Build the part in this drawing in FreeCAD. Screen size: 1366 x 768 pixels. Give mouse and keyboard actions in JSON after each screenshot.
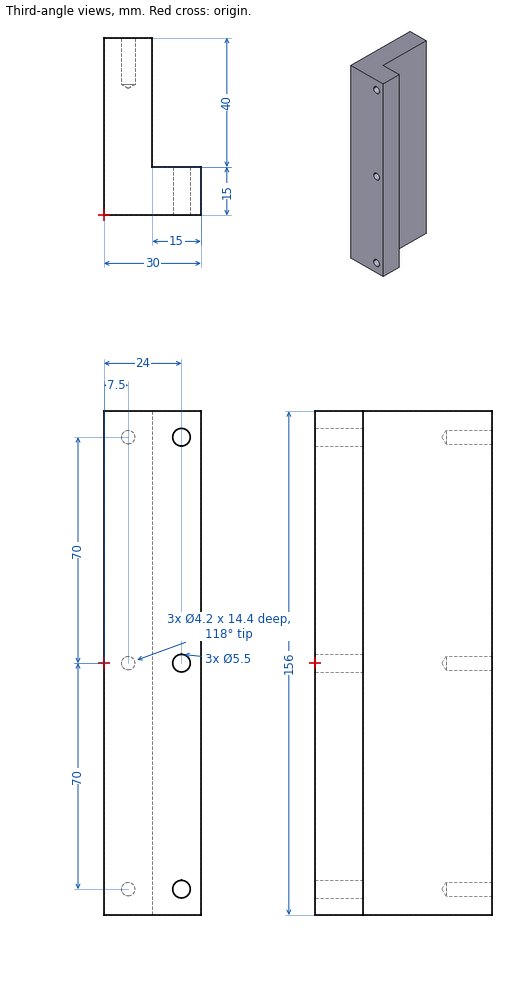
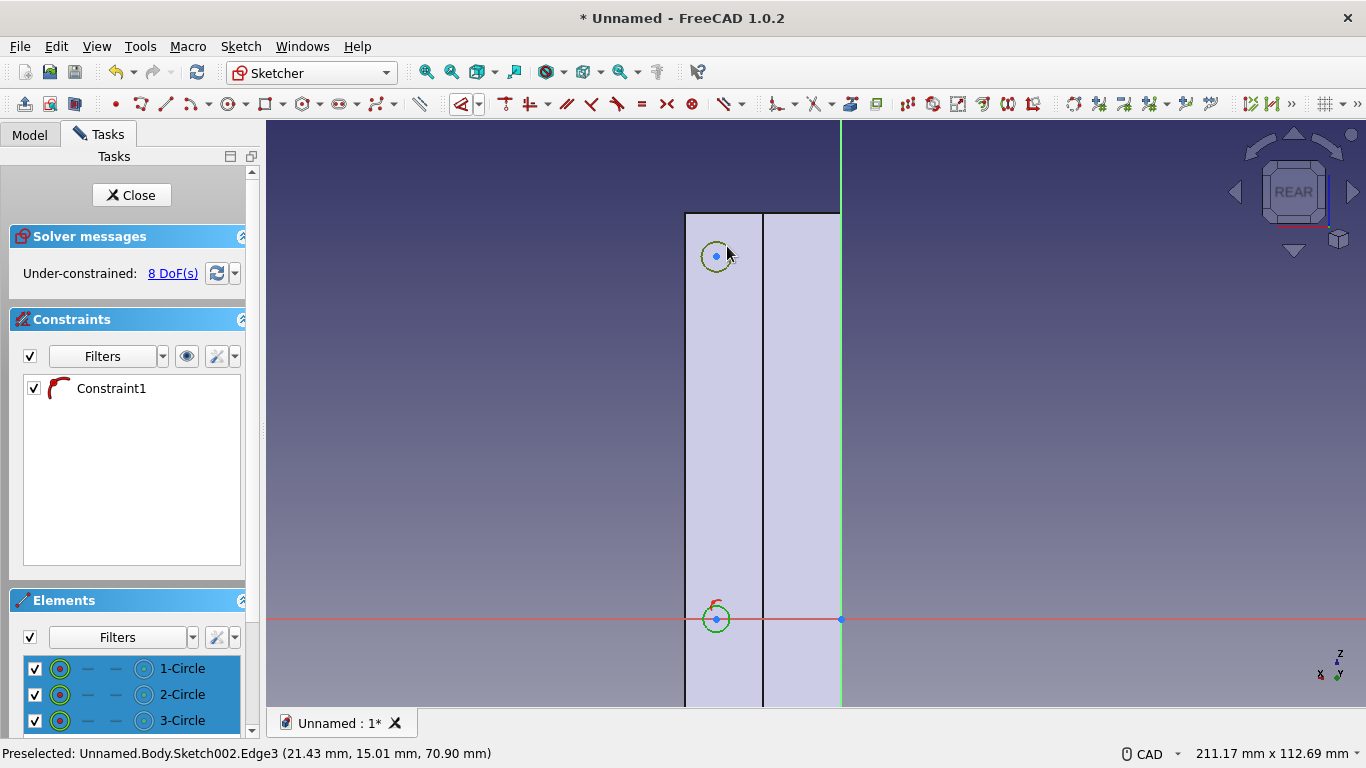
{"action": "key", "text": "e"}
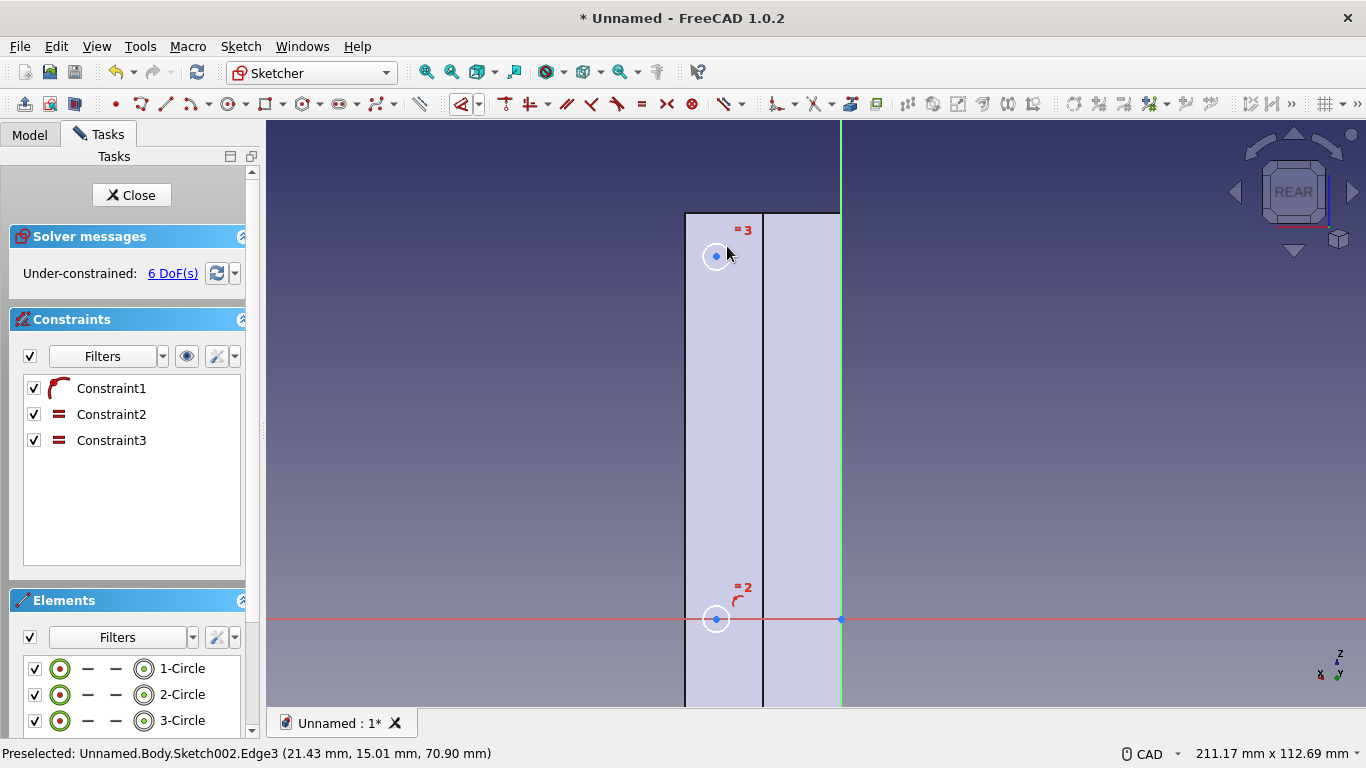
{"action": "left_click", "coordinate": [716, 619]}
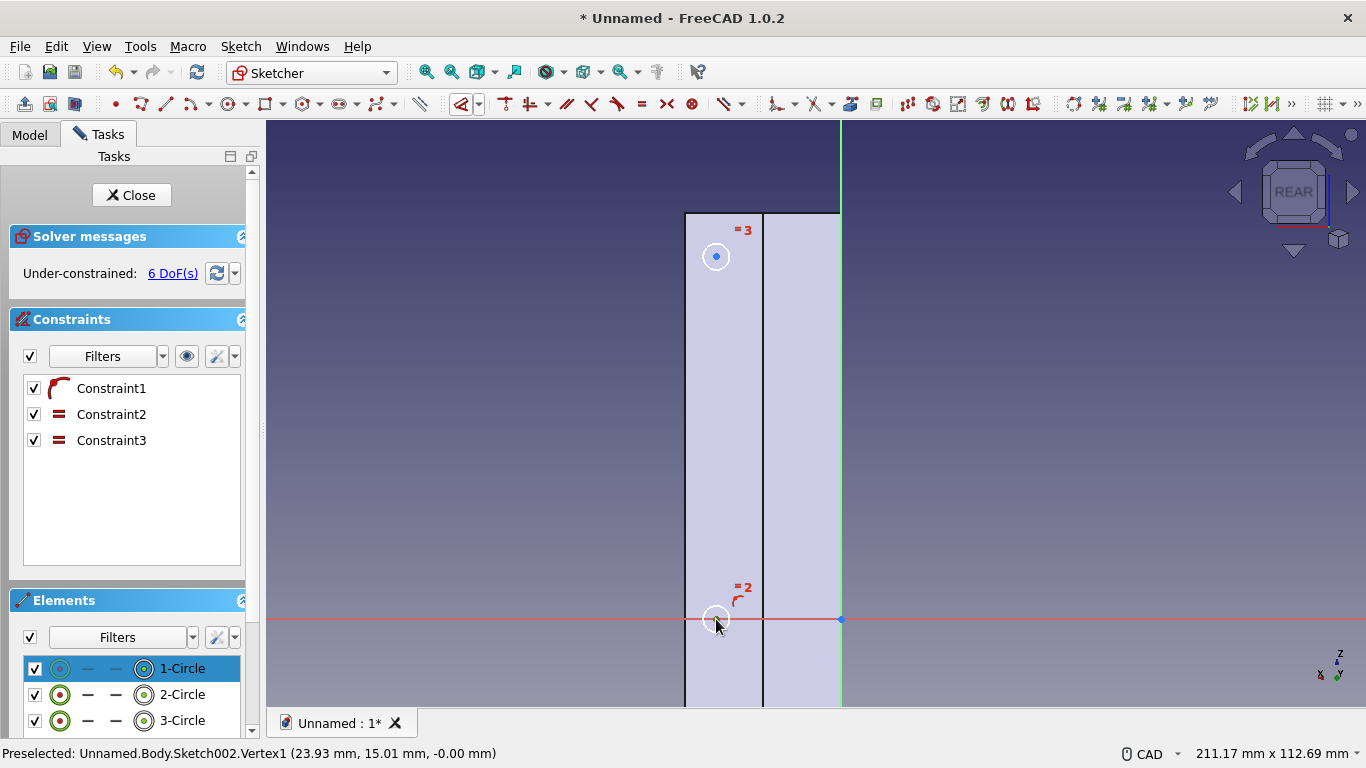
{"action": "scroll", "coordinate": [728, 246], "scroll_direction": "down", "scroll_amount": 4}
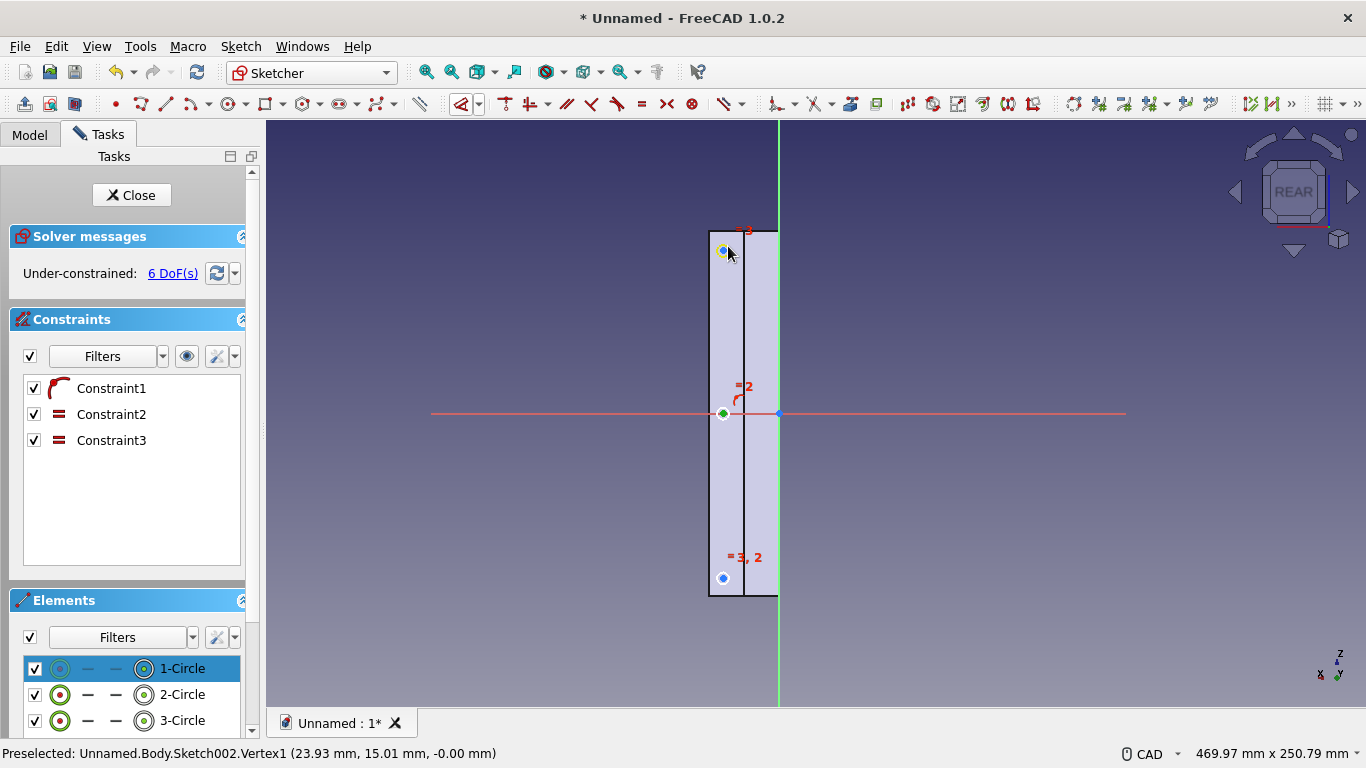
{"action": "left_click", "coordinate": [723, 578]}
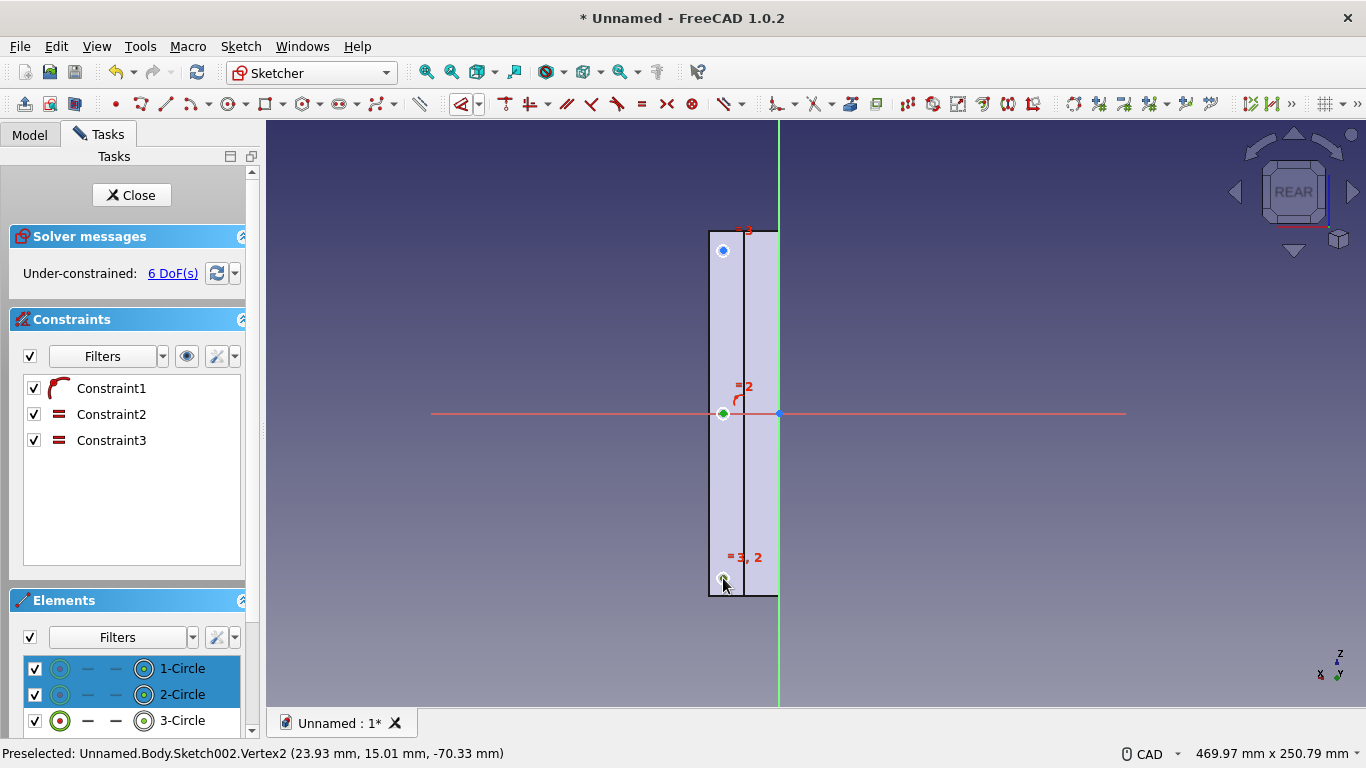
{"action": "left_click", "coordinate": [548, 104]}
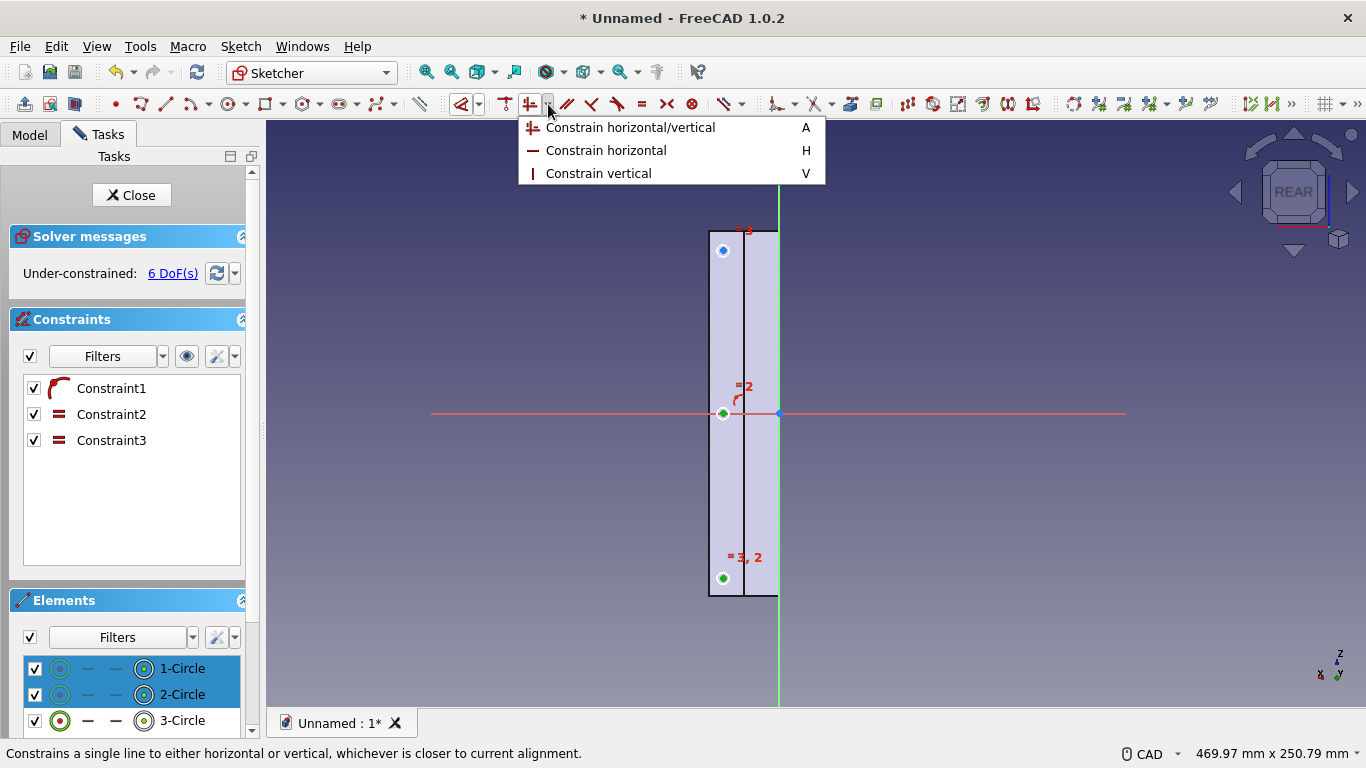
{"action": "left_click", "coordinate": [672, 174]}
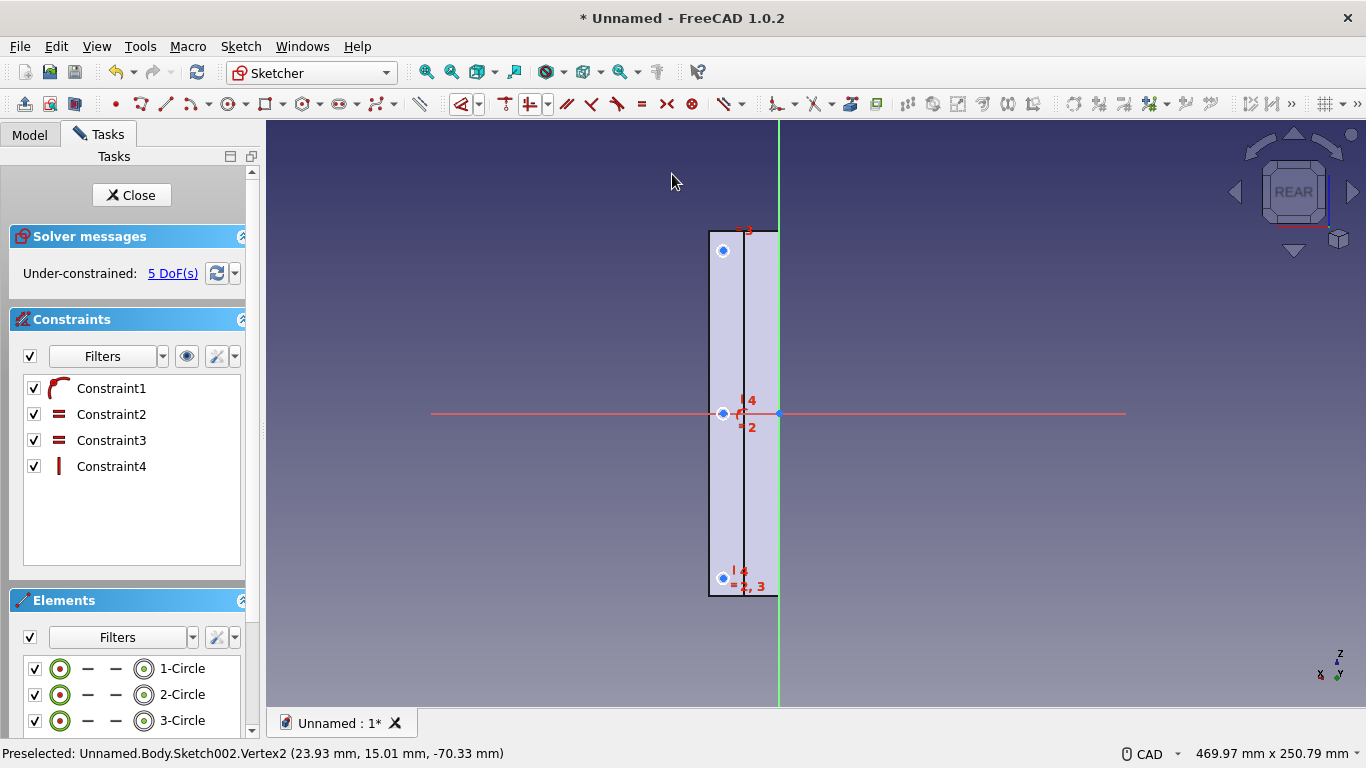
{"action": "left_click", "coordinate": [723, 414]}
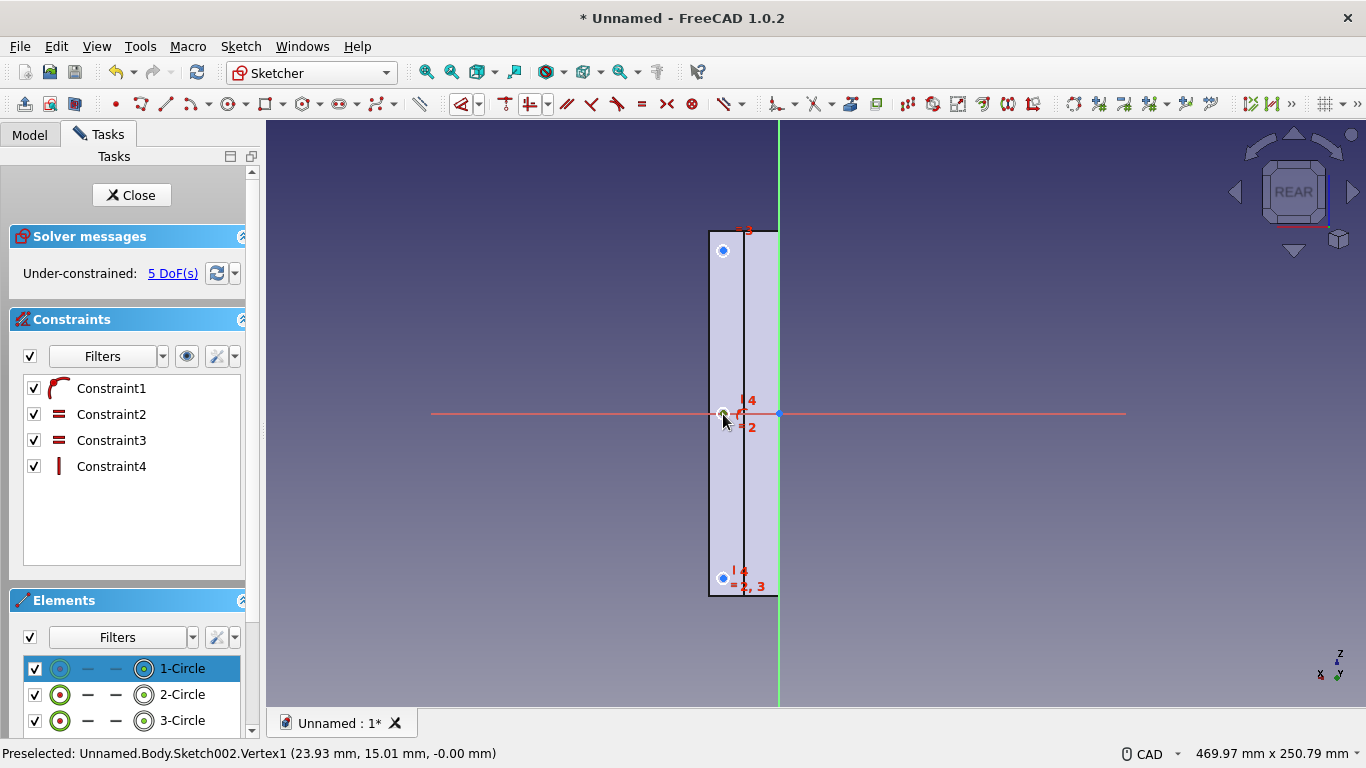
{"action": "left_click", "coordinate": [723, 251]}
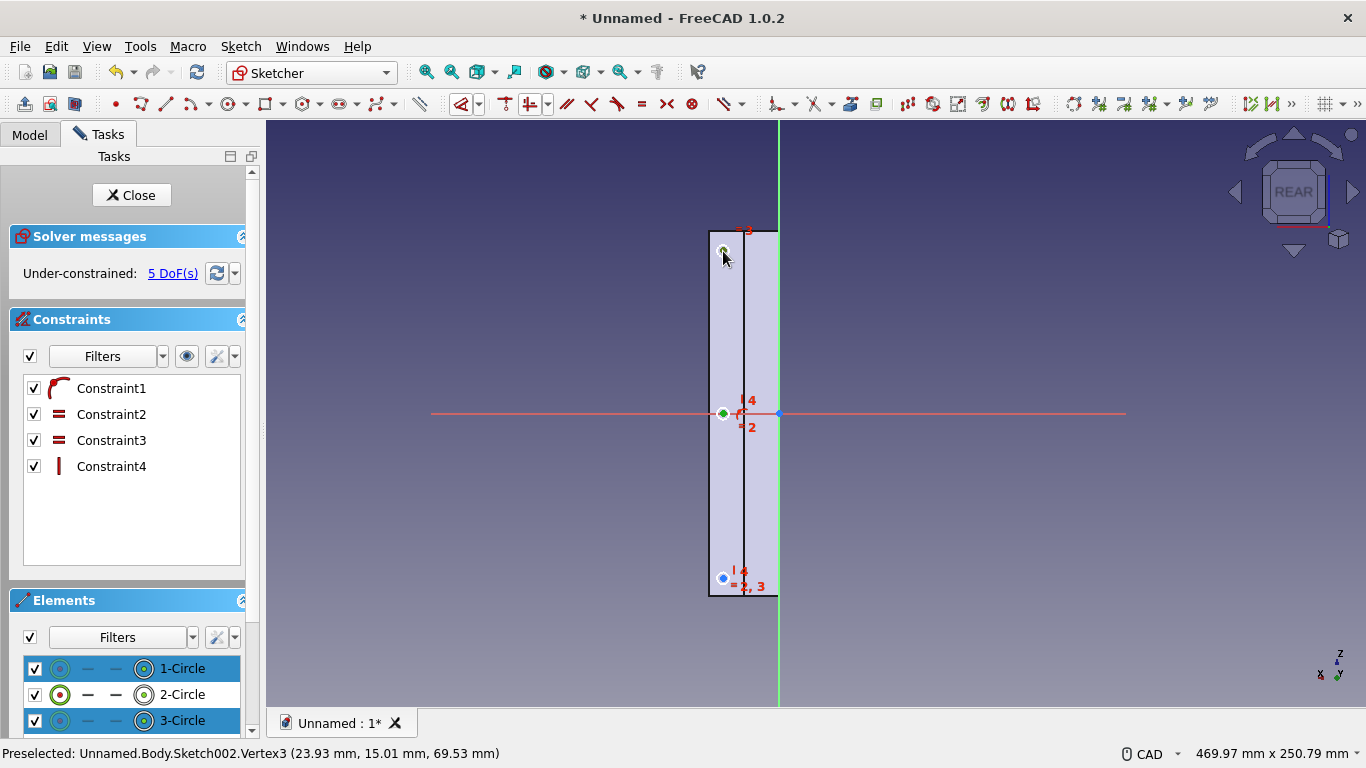
{"action": "key", "text": "v"}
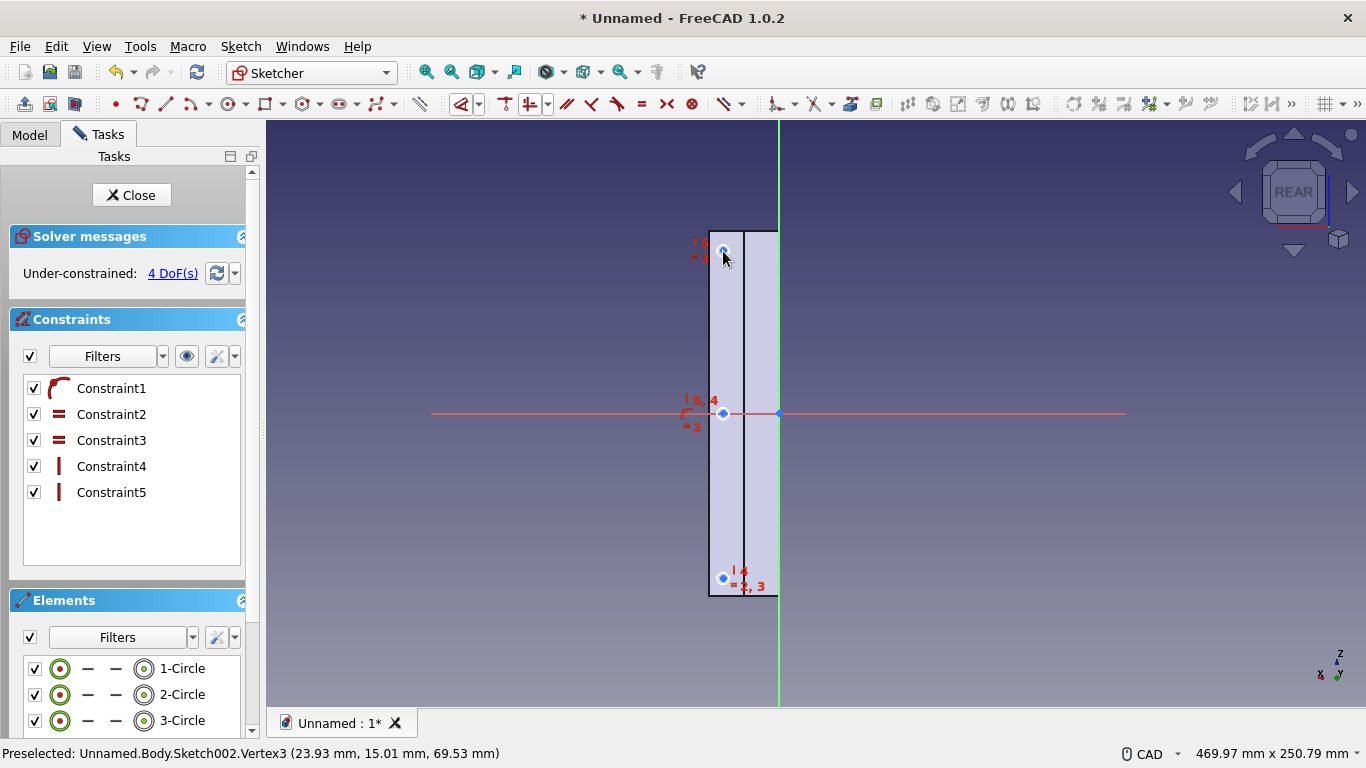
{"action": "scroll", "coordinate": [717, 414], "scroll_direction": "up", "scroll_amount": 6}